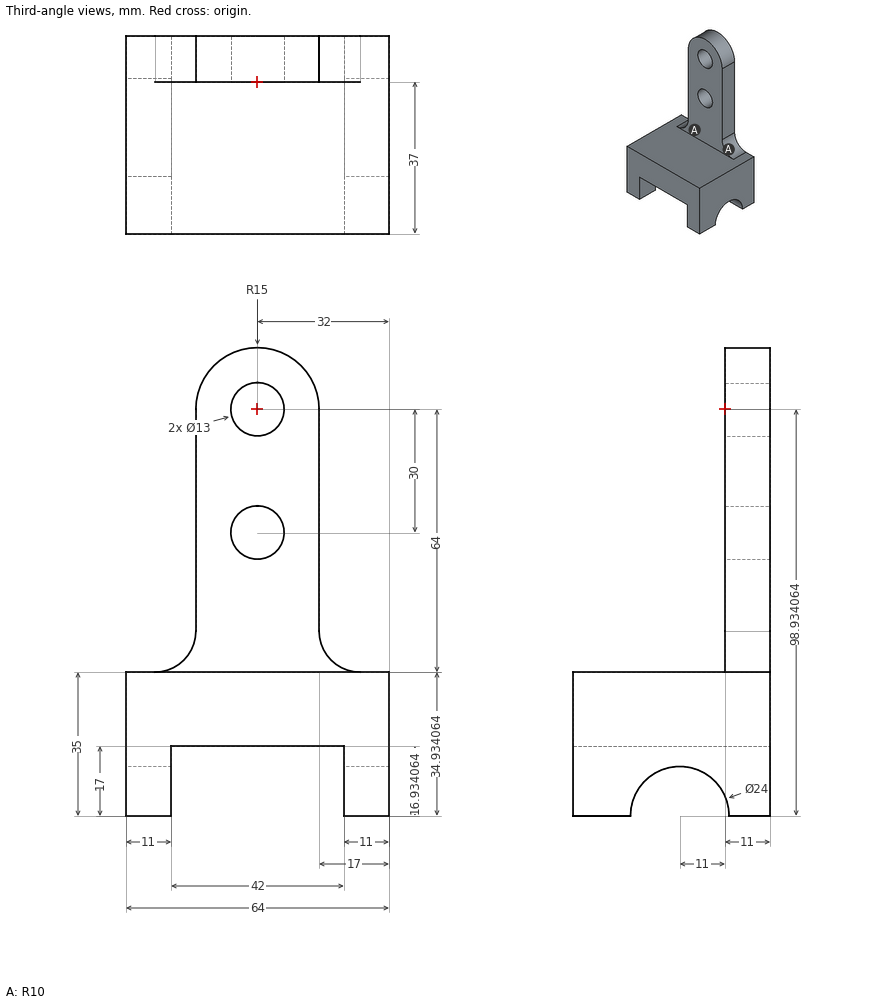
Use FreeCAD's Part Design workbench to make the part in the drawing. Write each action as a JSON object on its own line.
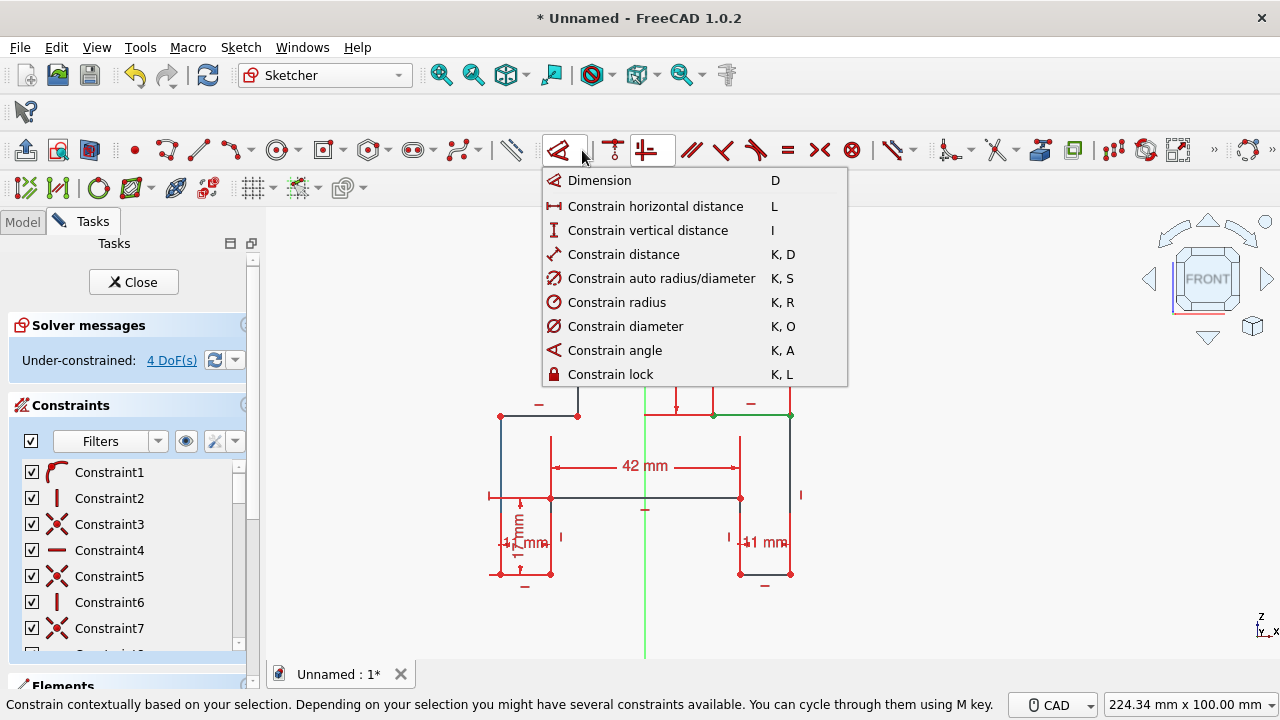
{"action": "left_click", "coordinate": [695, 230]}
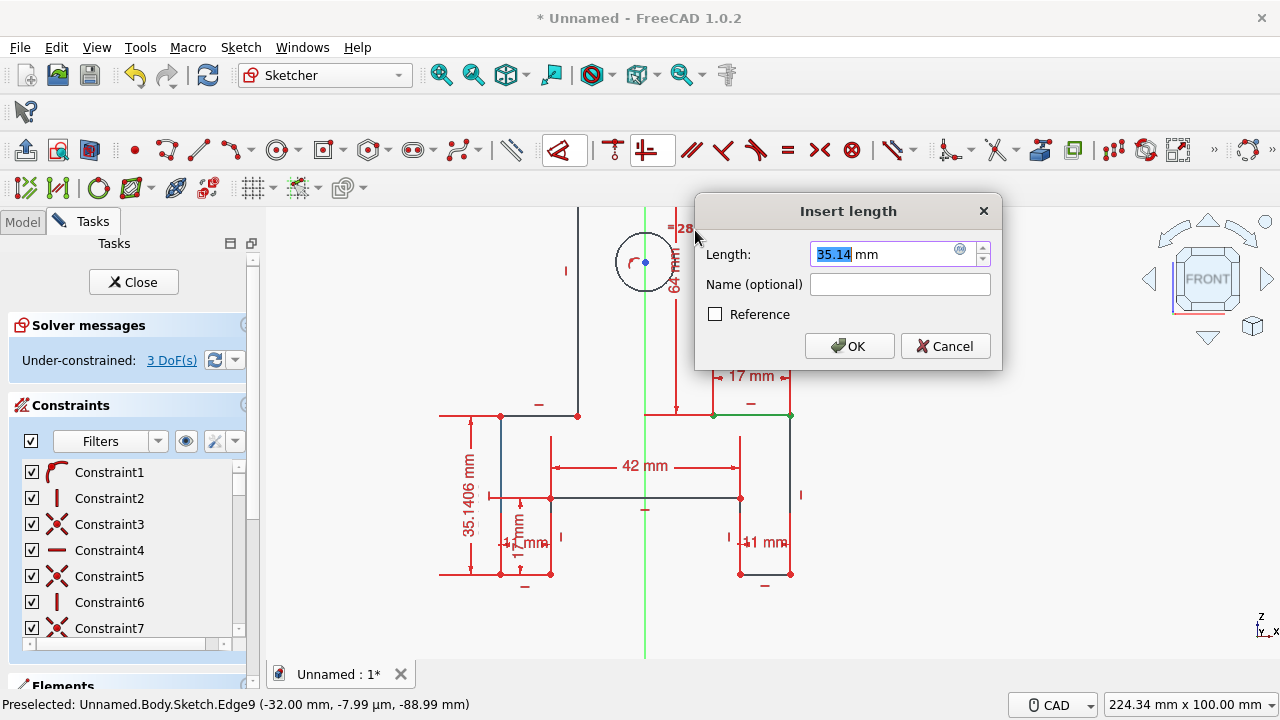
{"action": "type", "text": "35"}
{"action": "key", "text": "Return"}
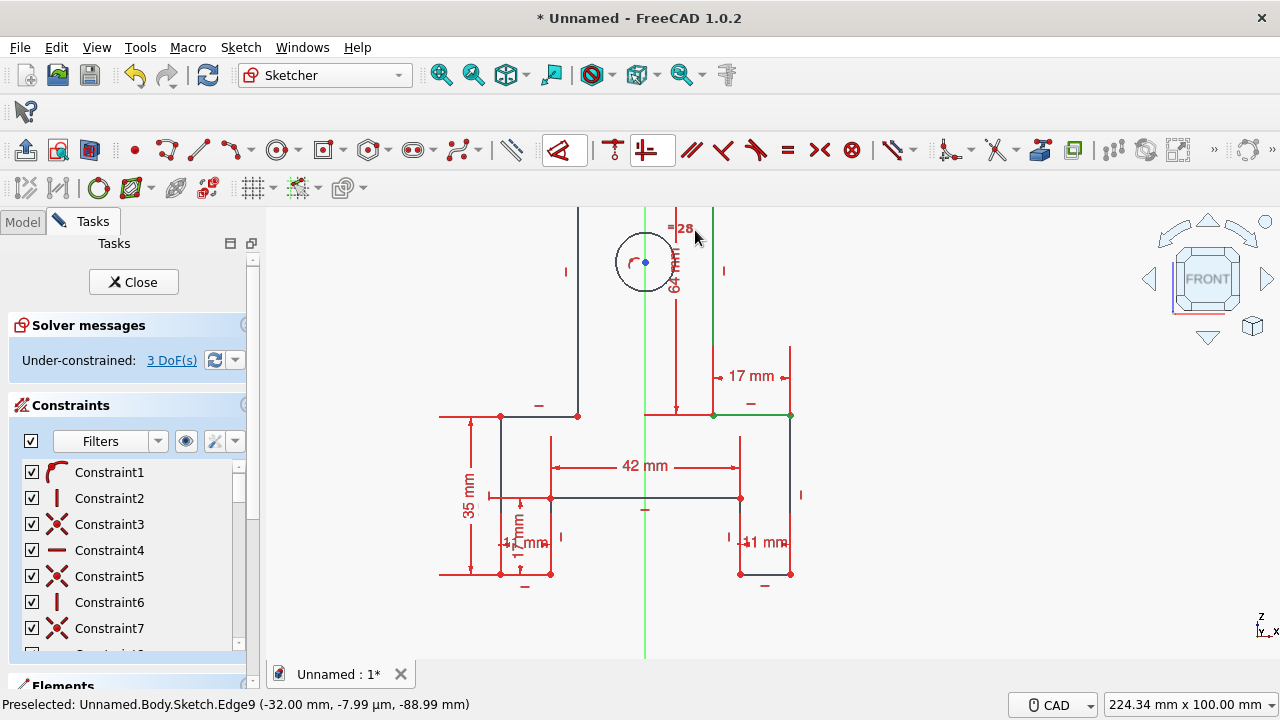
{"action": "left_click", "coordinate": [578, 329]}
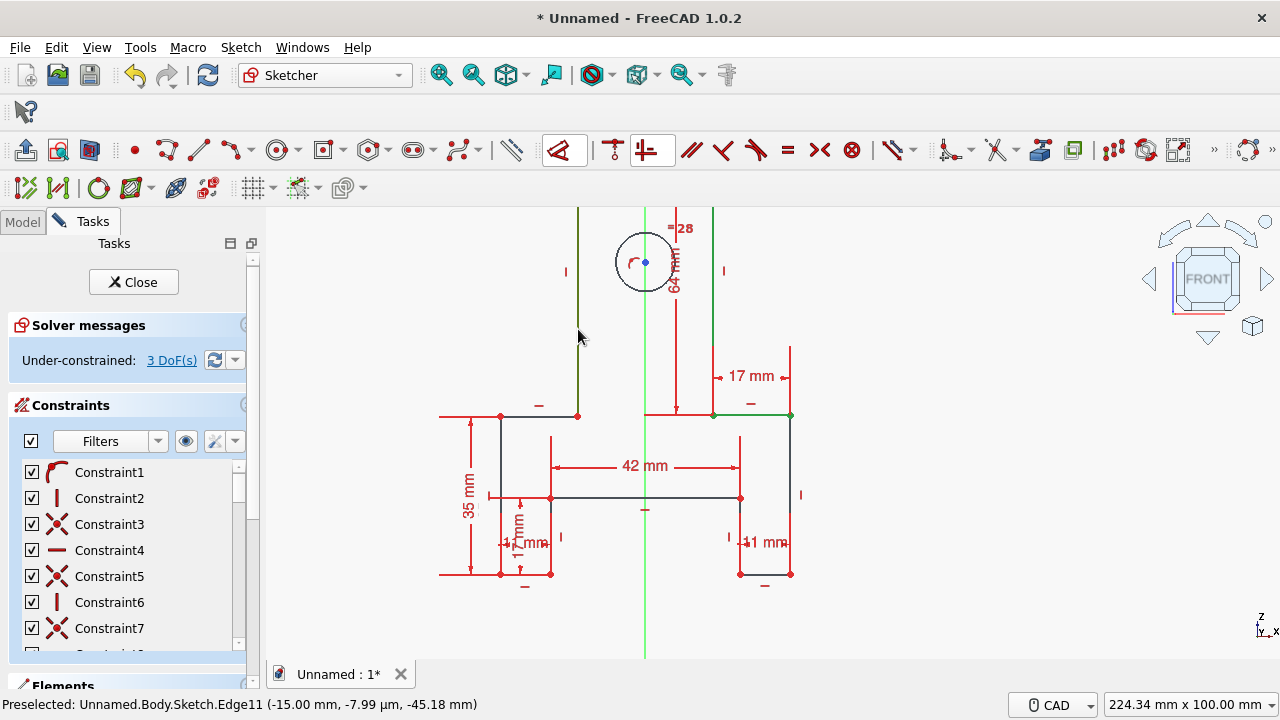
{"action": "left_click", "coordinate": [582, 150]}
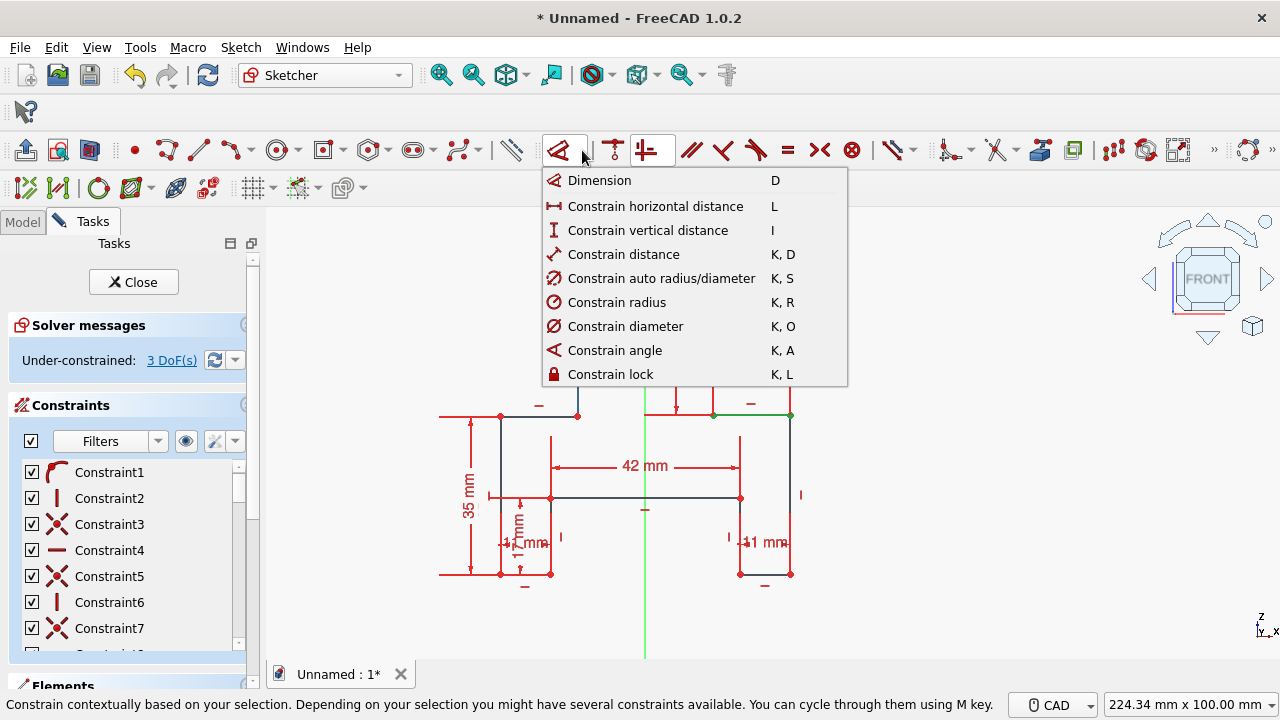
{"action": "left_click", "coordinate": [695, 230]}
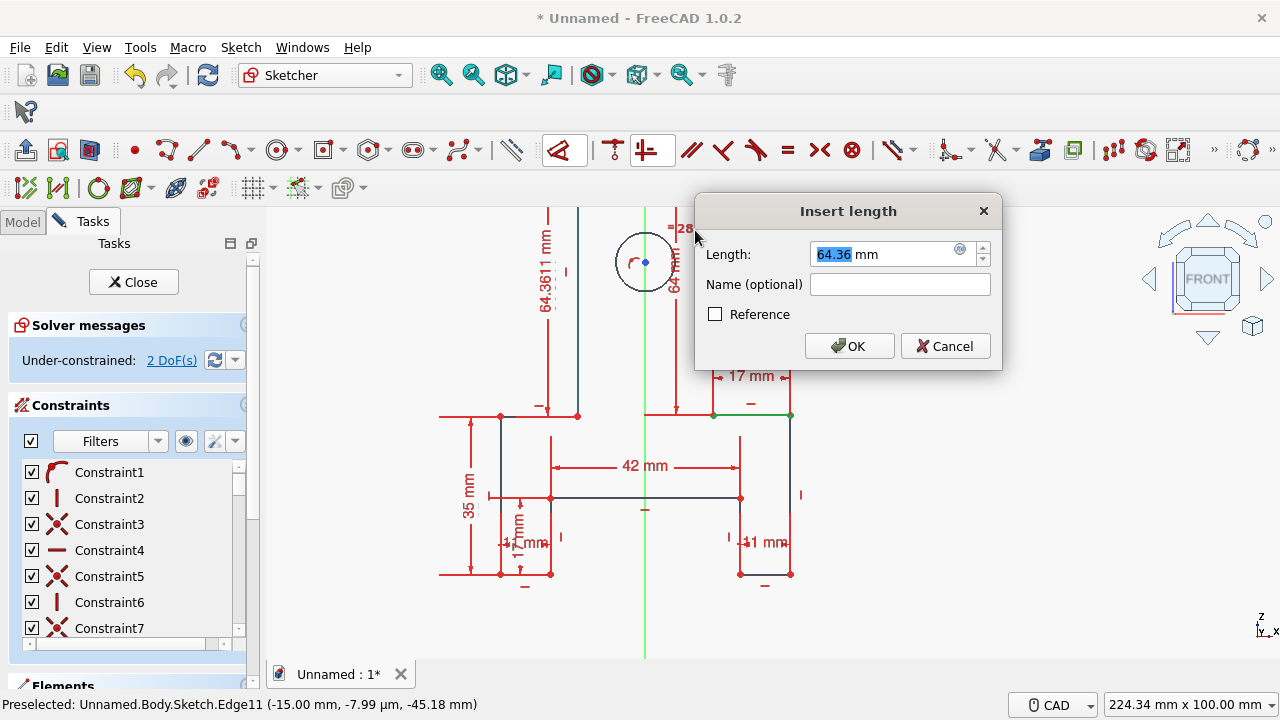
{"action": "type", "text": "64"}
{"action": "key", "text": "Return"}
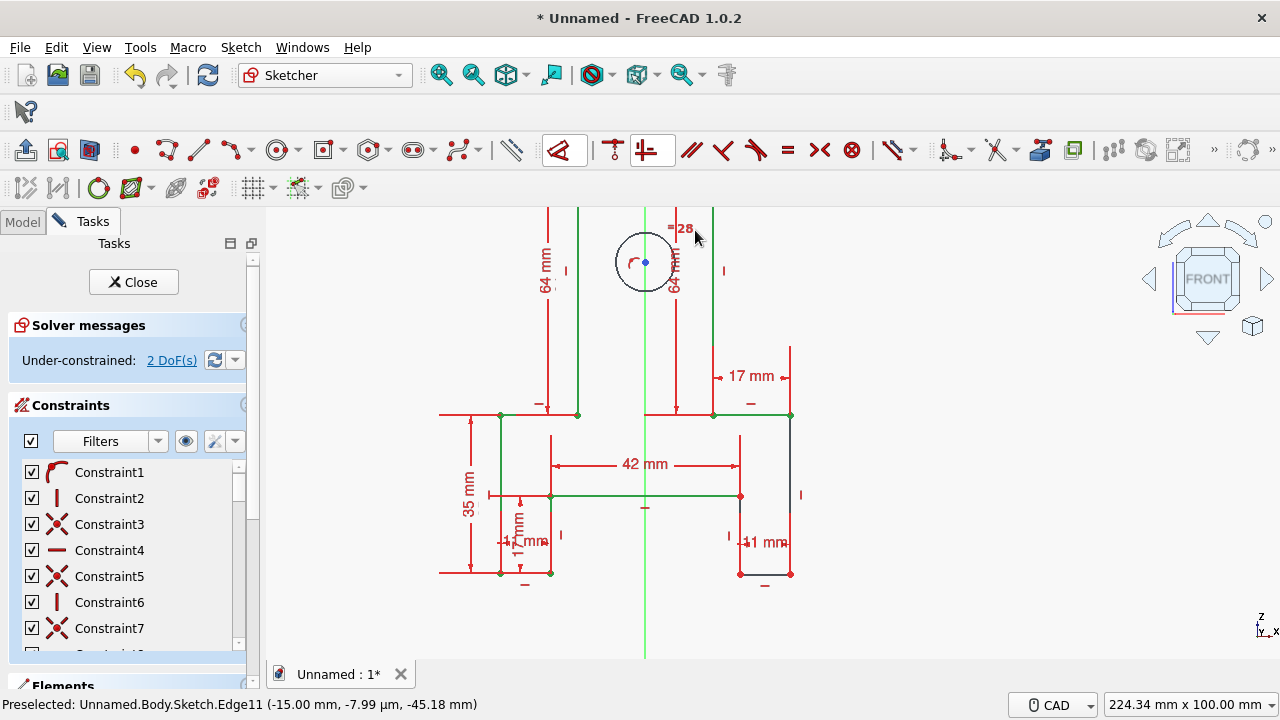
{"action": "left_click", "coordinate": [645, 262]}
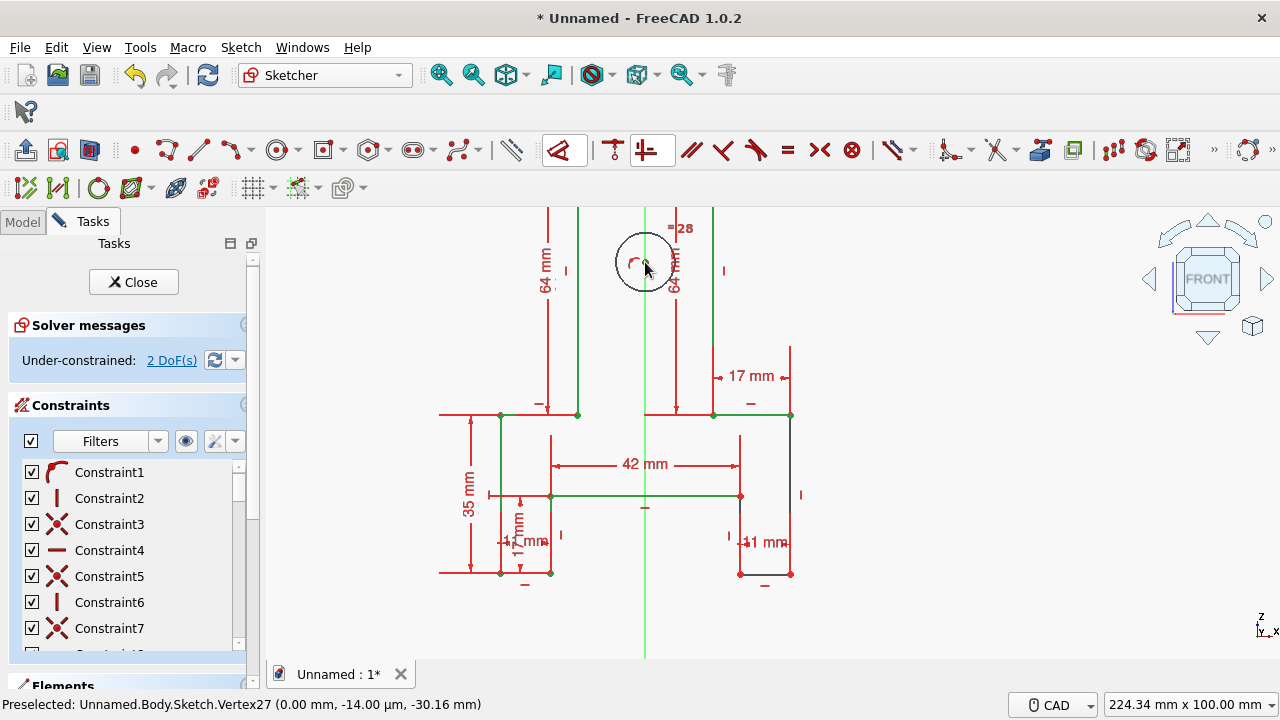
{"action": "left_click", "coordinate": [582, 150]}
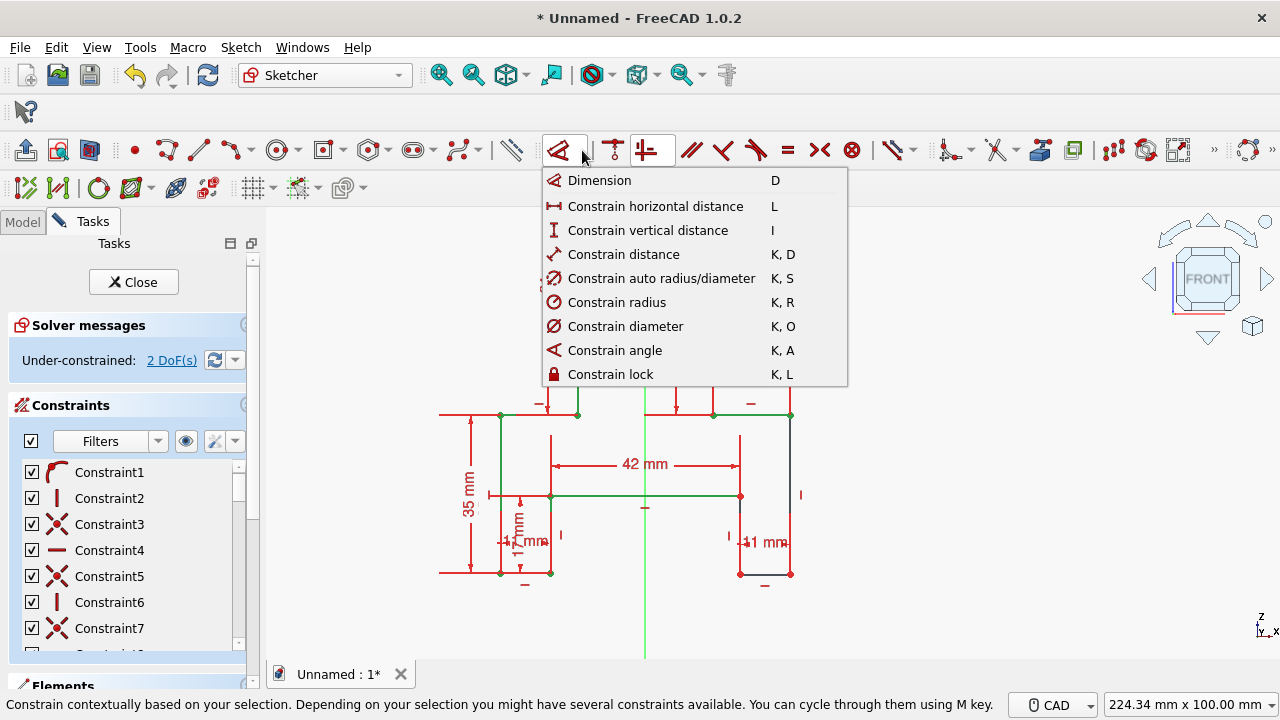
{"action": "left_click", "coordinate": [695, 230]}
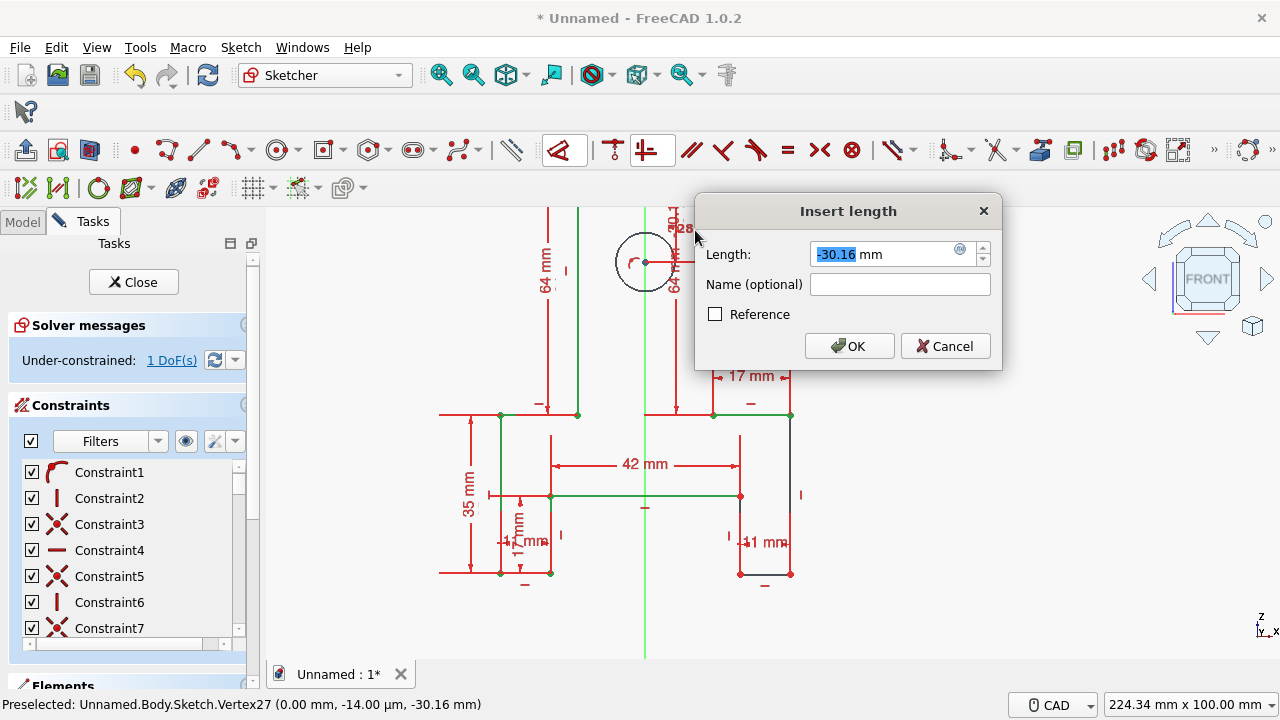
{"action": "type", "text": "-30"}
{"action": "key", "text": "Return"}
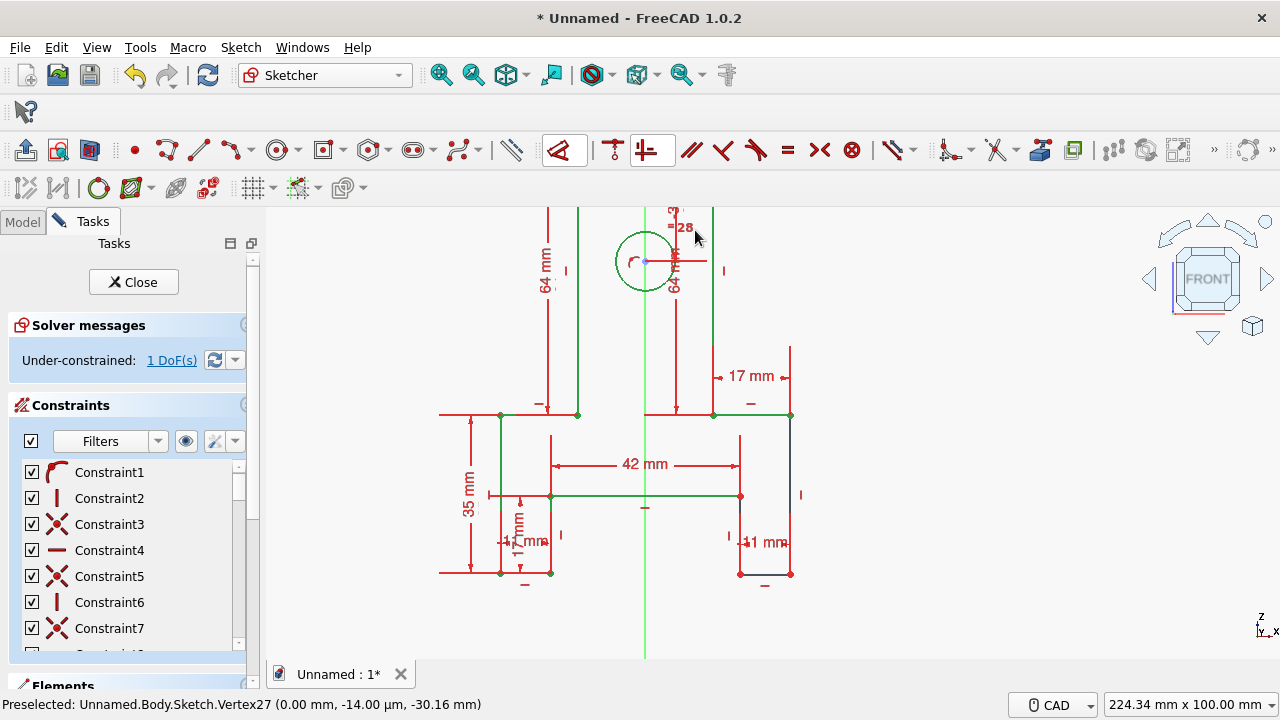
{"action": "left_click", "coordinate": [790, 463]}